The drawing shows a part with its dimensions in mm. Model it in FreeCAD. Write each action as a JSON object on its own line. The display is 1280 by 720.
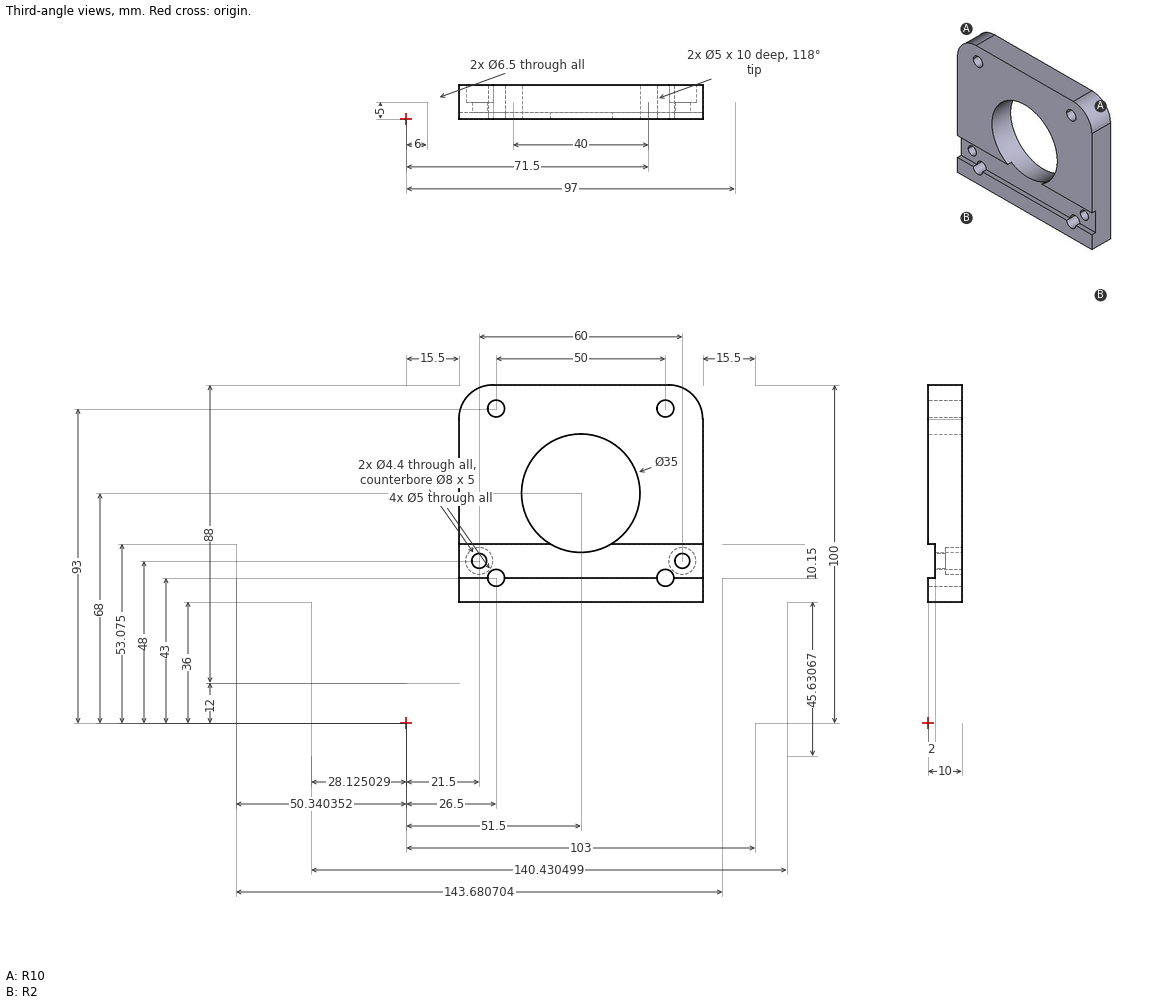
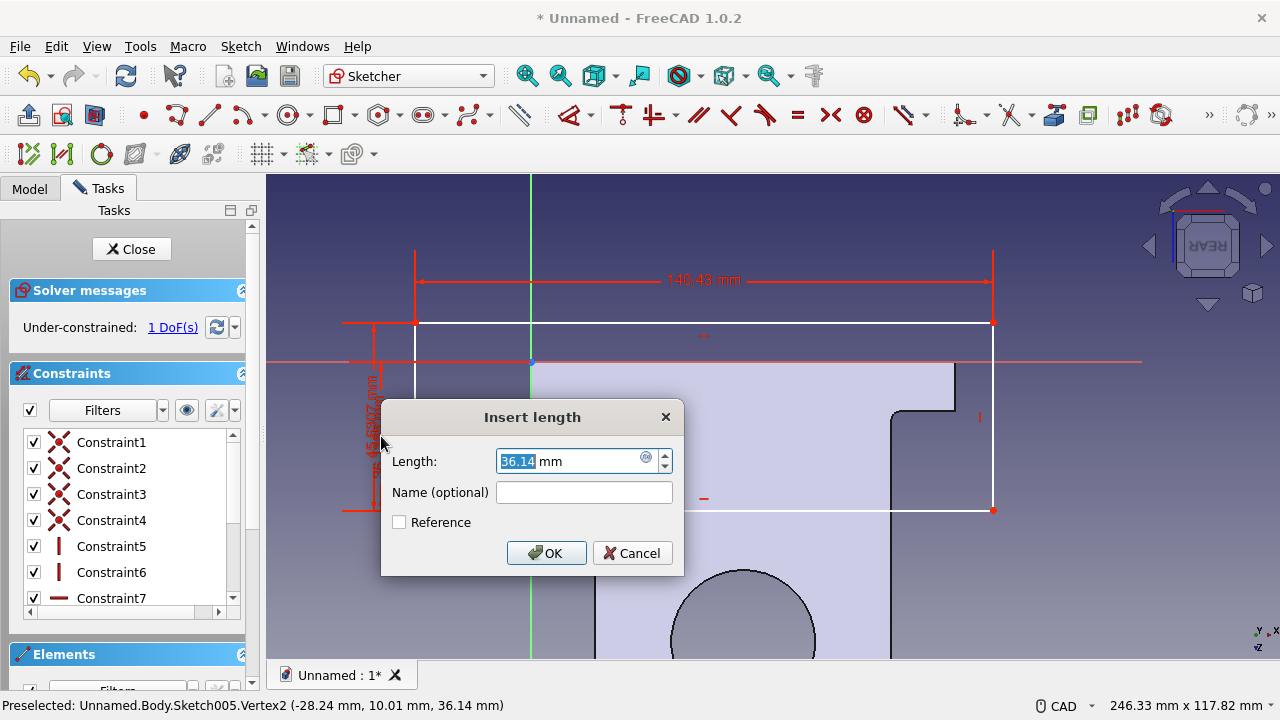
{"action": "type", "text": "36"}
{"action": "key", "text": "Return"}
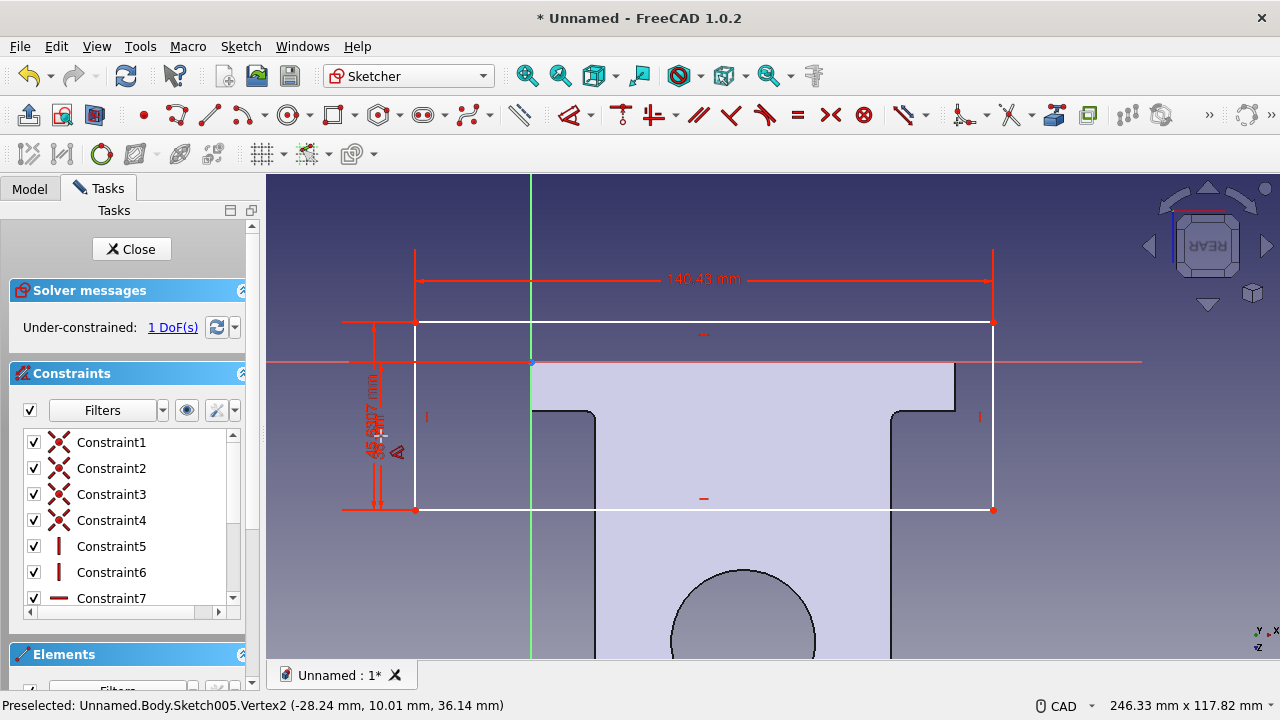
{"action": "left_click", "coordinate": [415, 322]}
{"action": "left_click", "coordinate": [473, 288]}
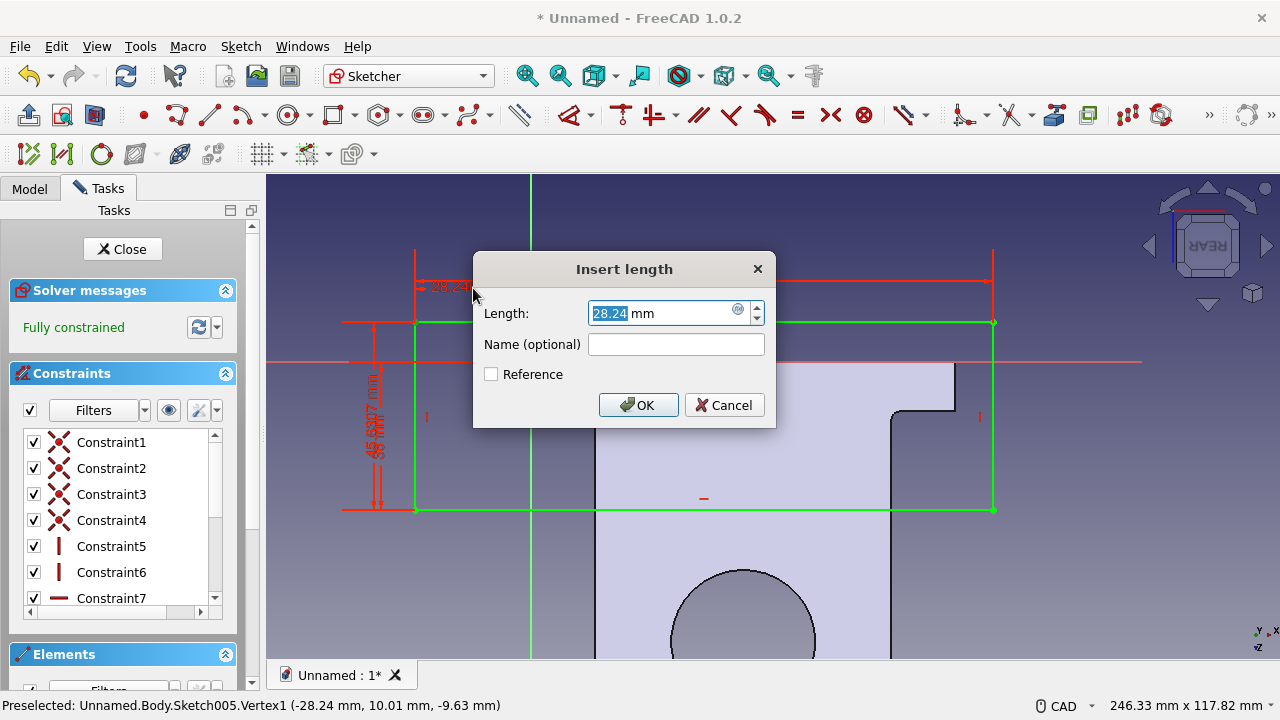
{"action": "type", "text": "28.125029"}
{"action": "key", "text": "Return"}
{"action": "key", "text": "Escape"}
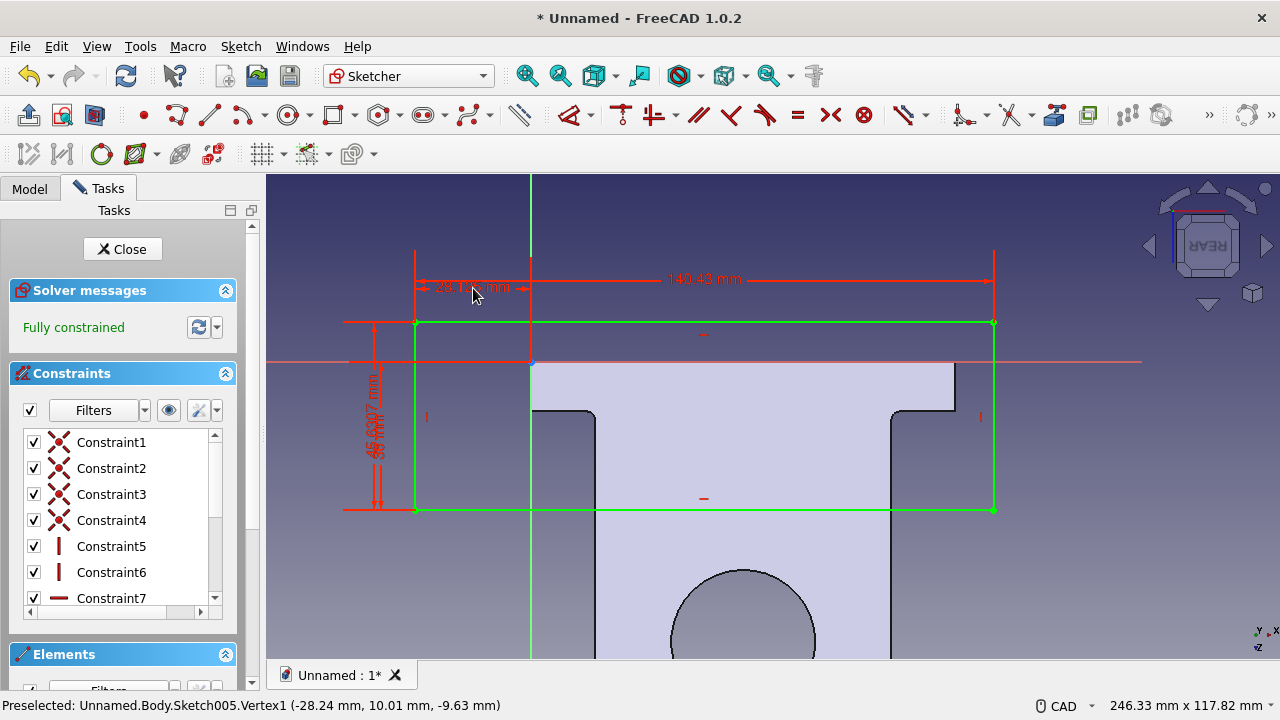
{"action": "left_click", "coordinate": [123, 249]}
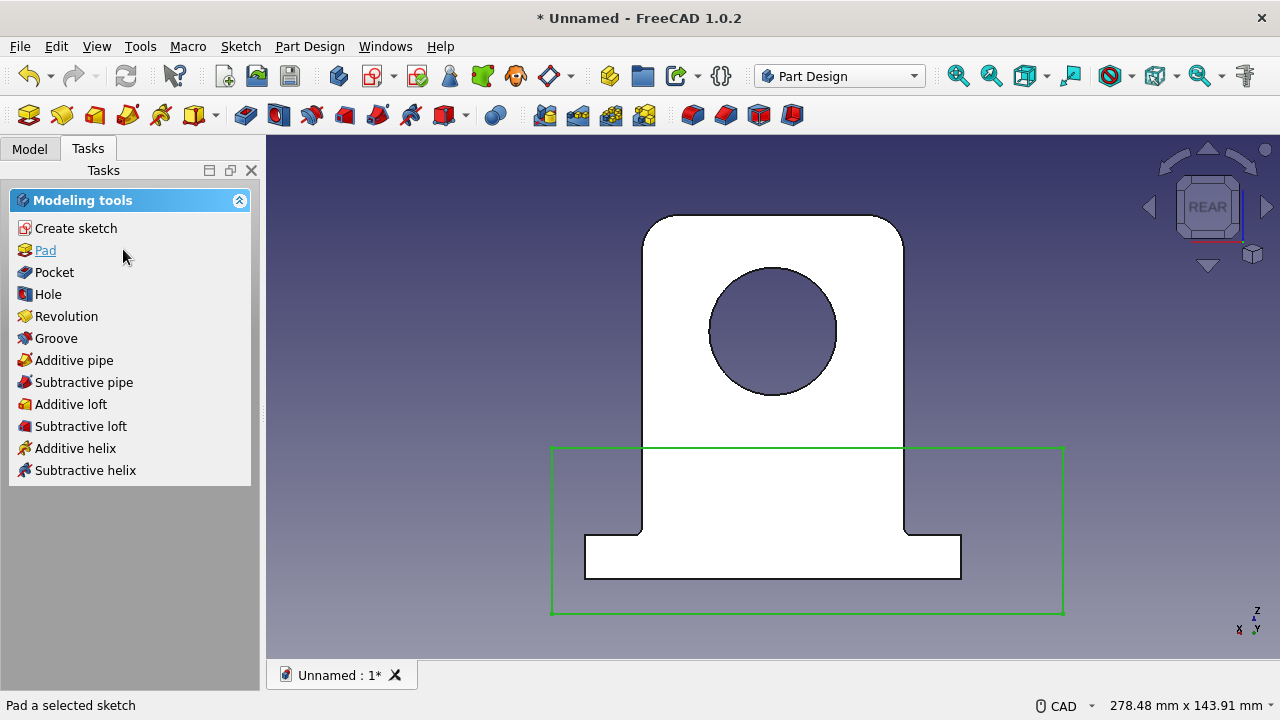
{"action": "left_click", "coordinate": [246, 116]}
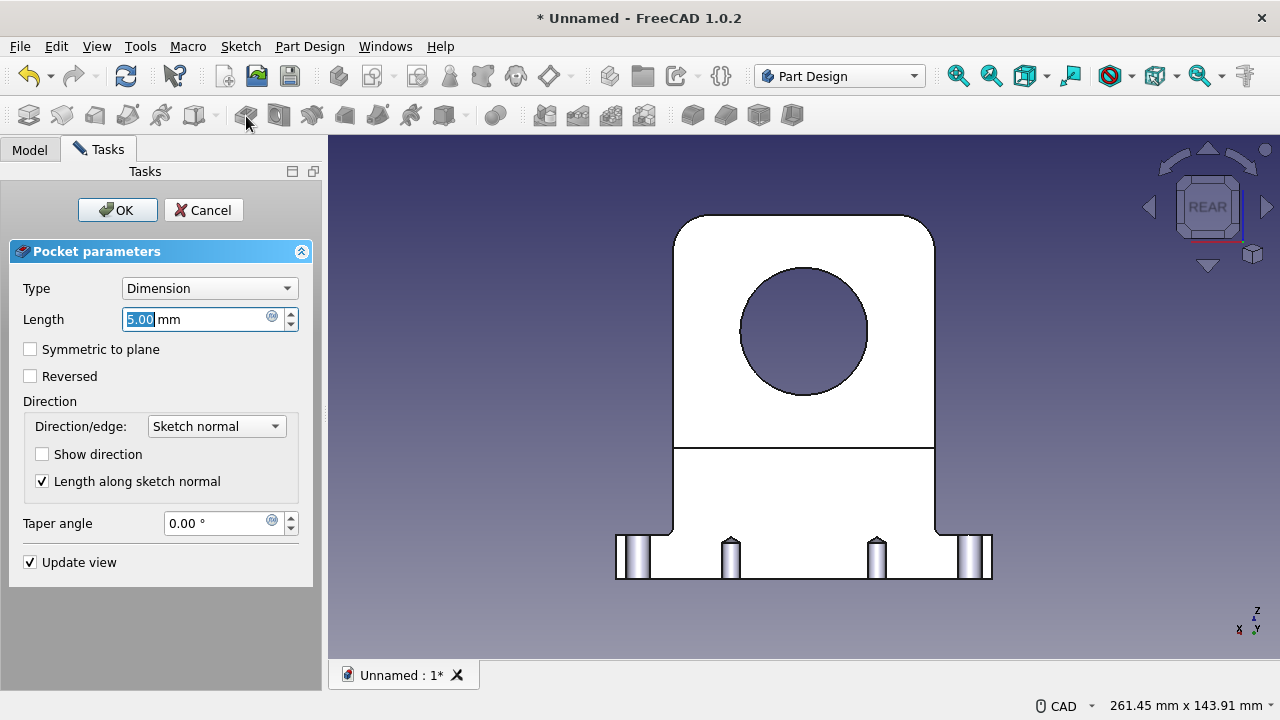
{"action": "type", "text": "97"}
{"action": "key", "text": "Tab"}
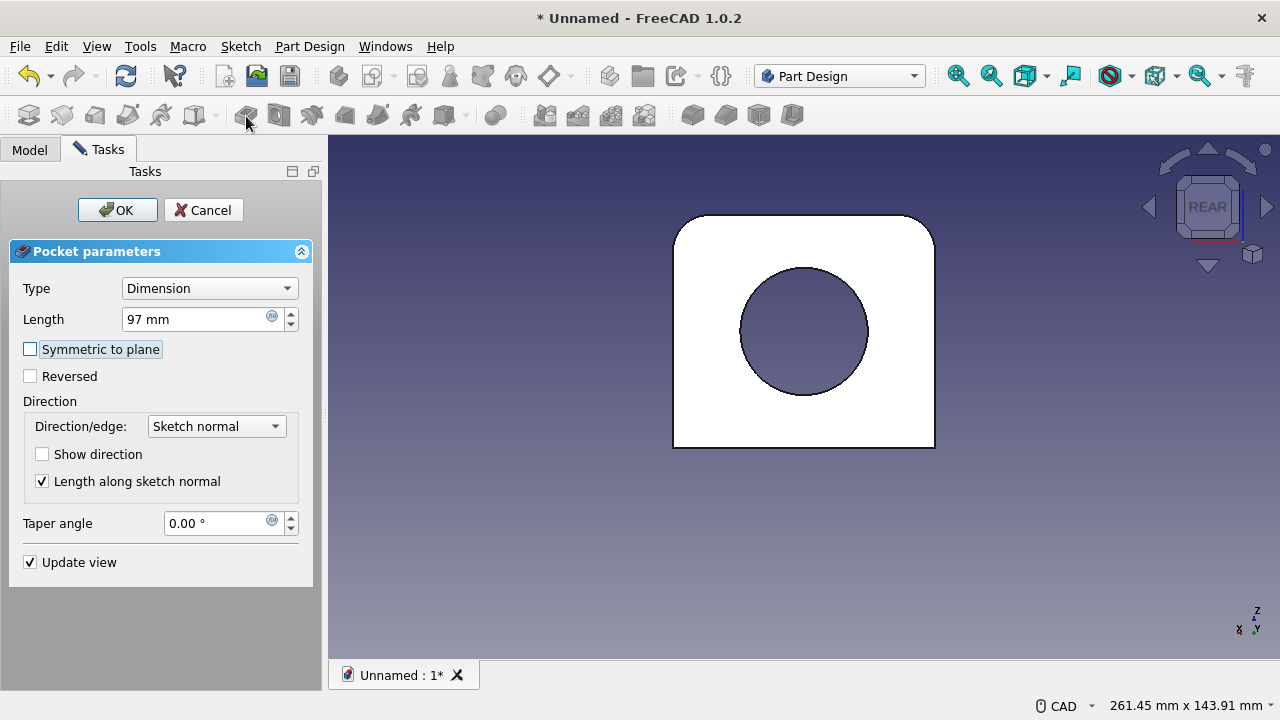
{"action": "left_click", "coordinate": [118, 210]}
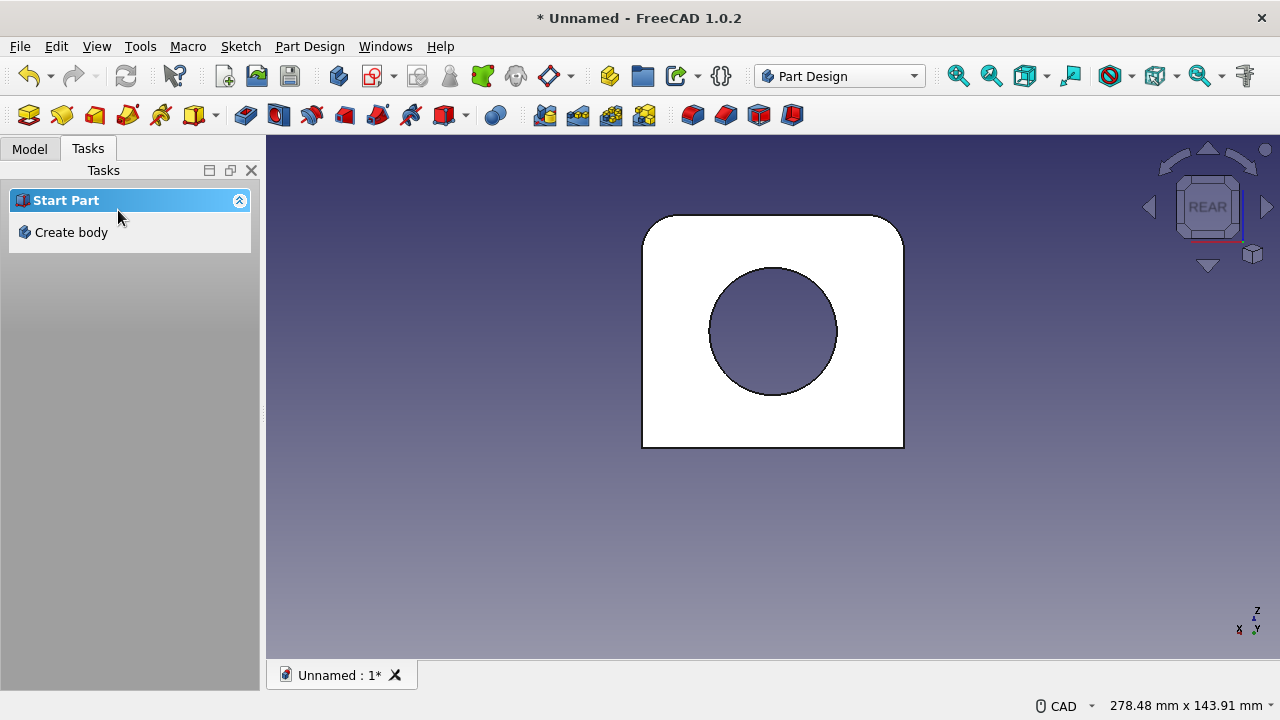
{"action": "key", "text": "v f"}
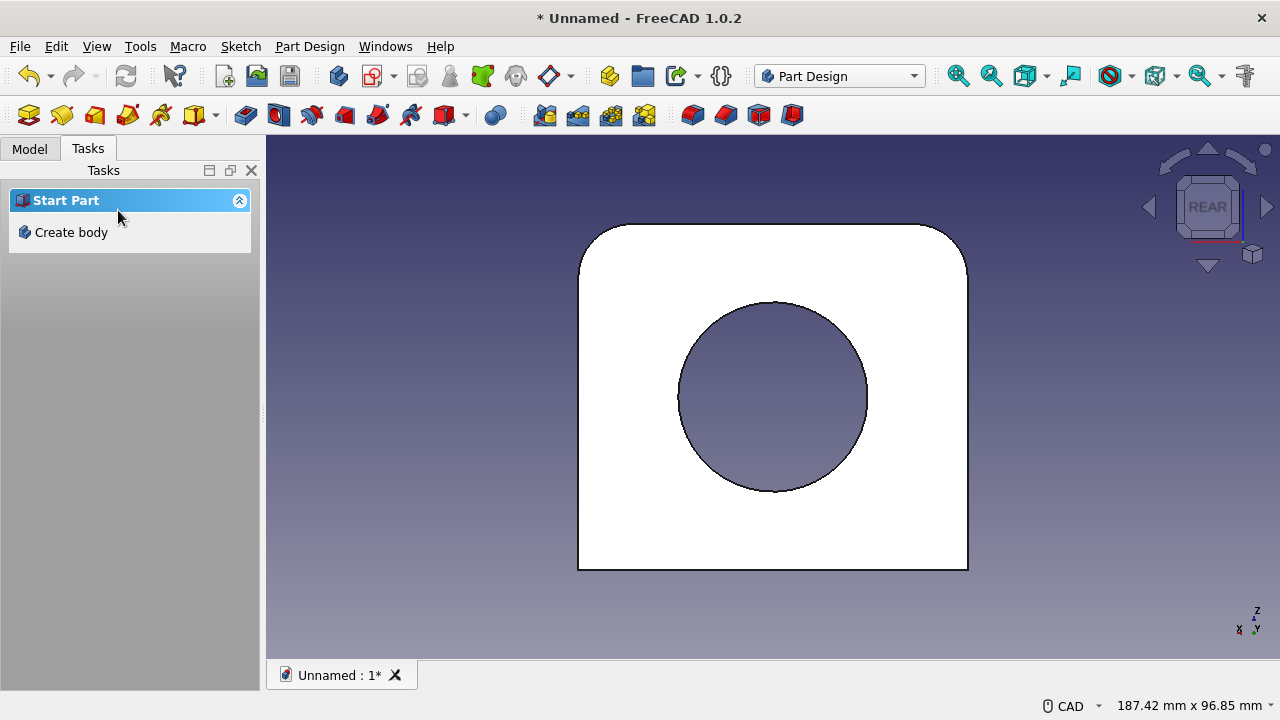
{"action": "left_click", "coordinate": [662, 297]}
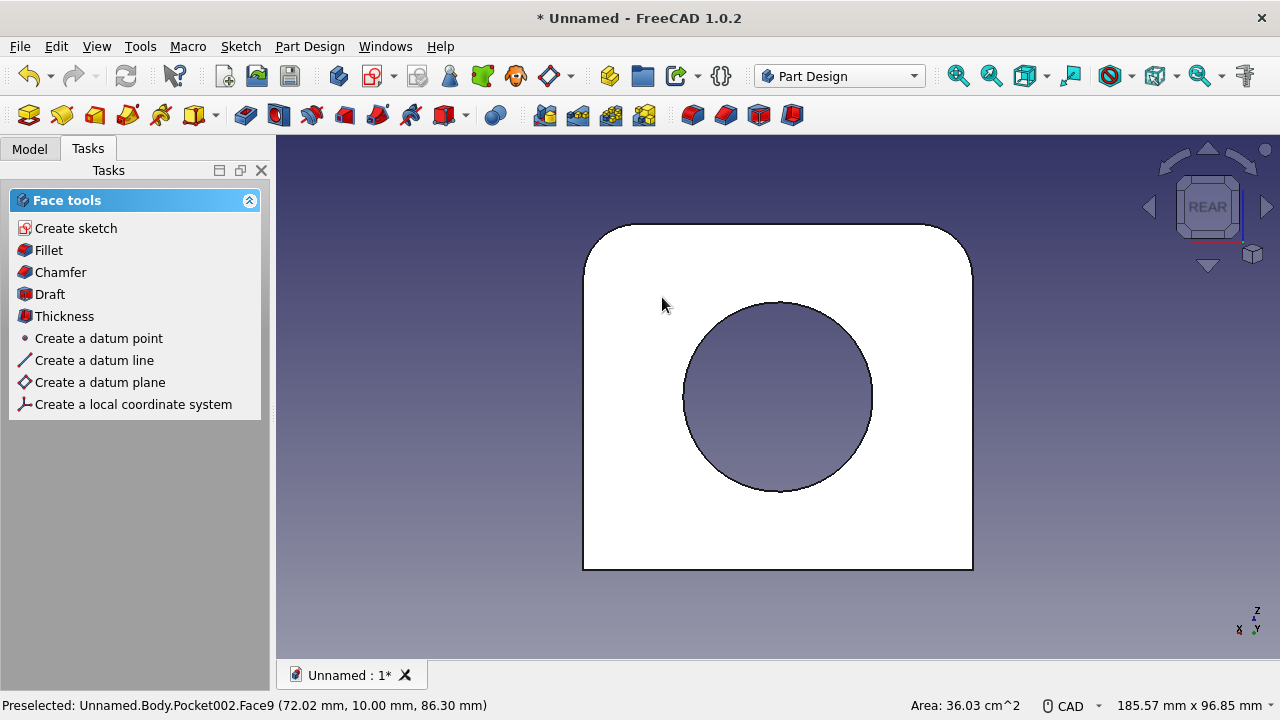
{"action": "left_click", "coordinate": [372, 76]}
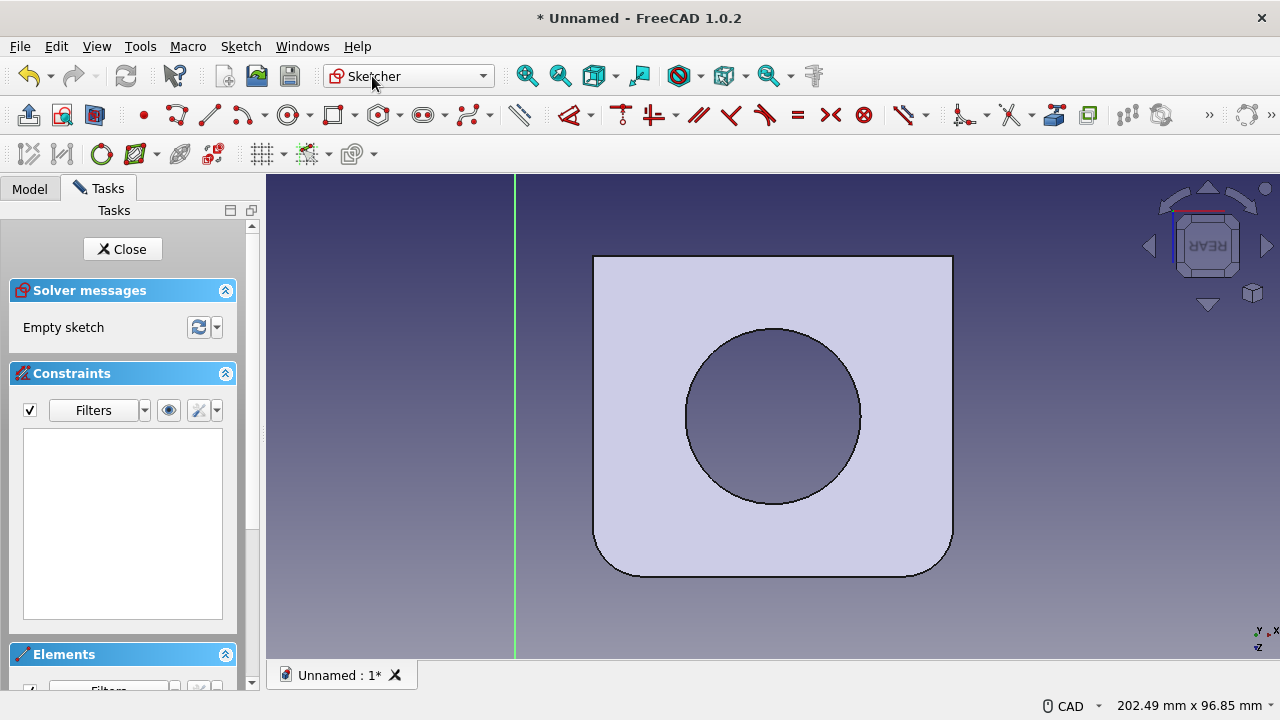
{"action": "scroll", "coordinate": [663, 631], "scroll_direction": "down", "scroll_amount": 2}